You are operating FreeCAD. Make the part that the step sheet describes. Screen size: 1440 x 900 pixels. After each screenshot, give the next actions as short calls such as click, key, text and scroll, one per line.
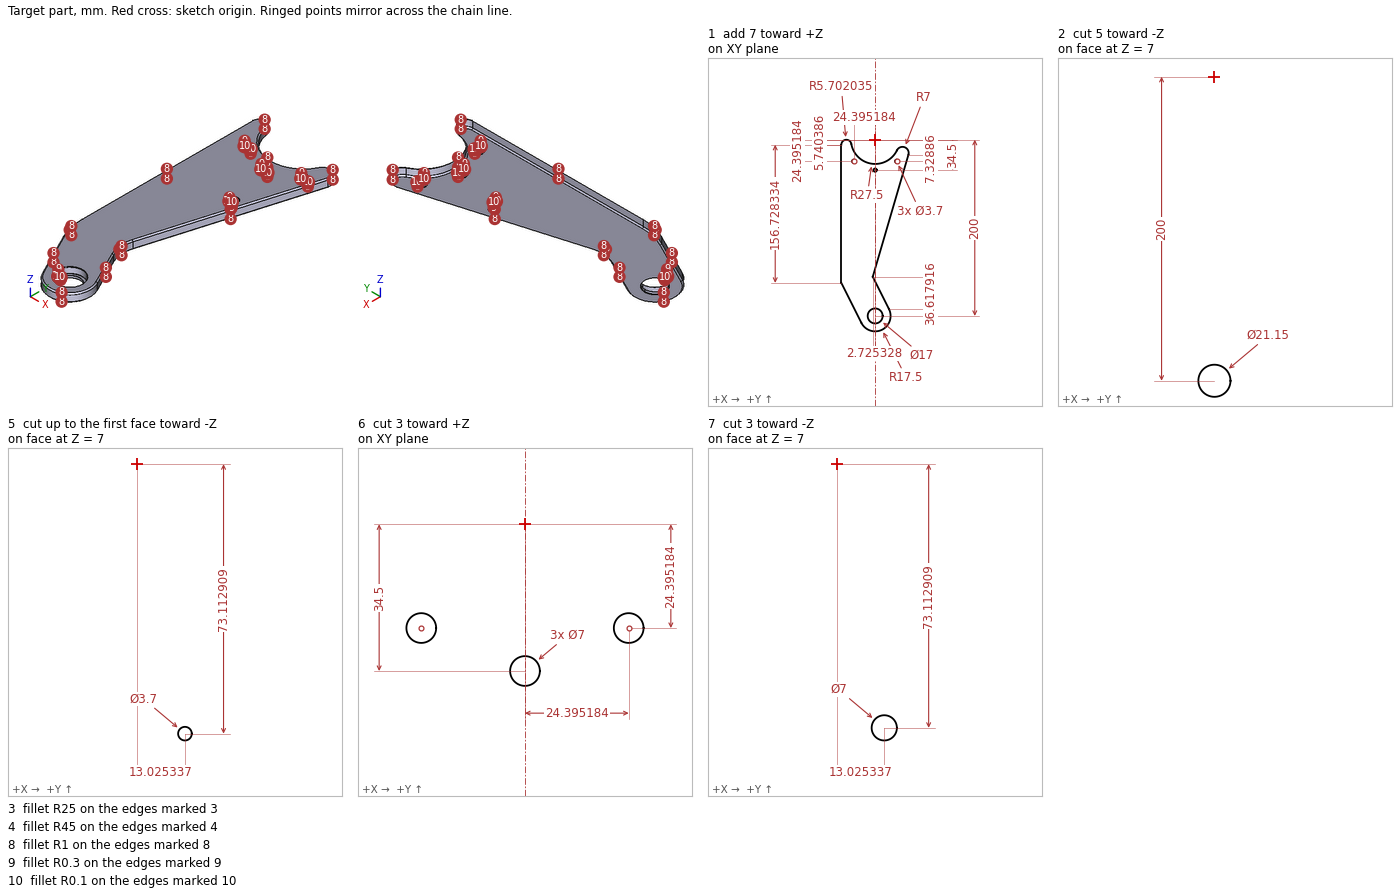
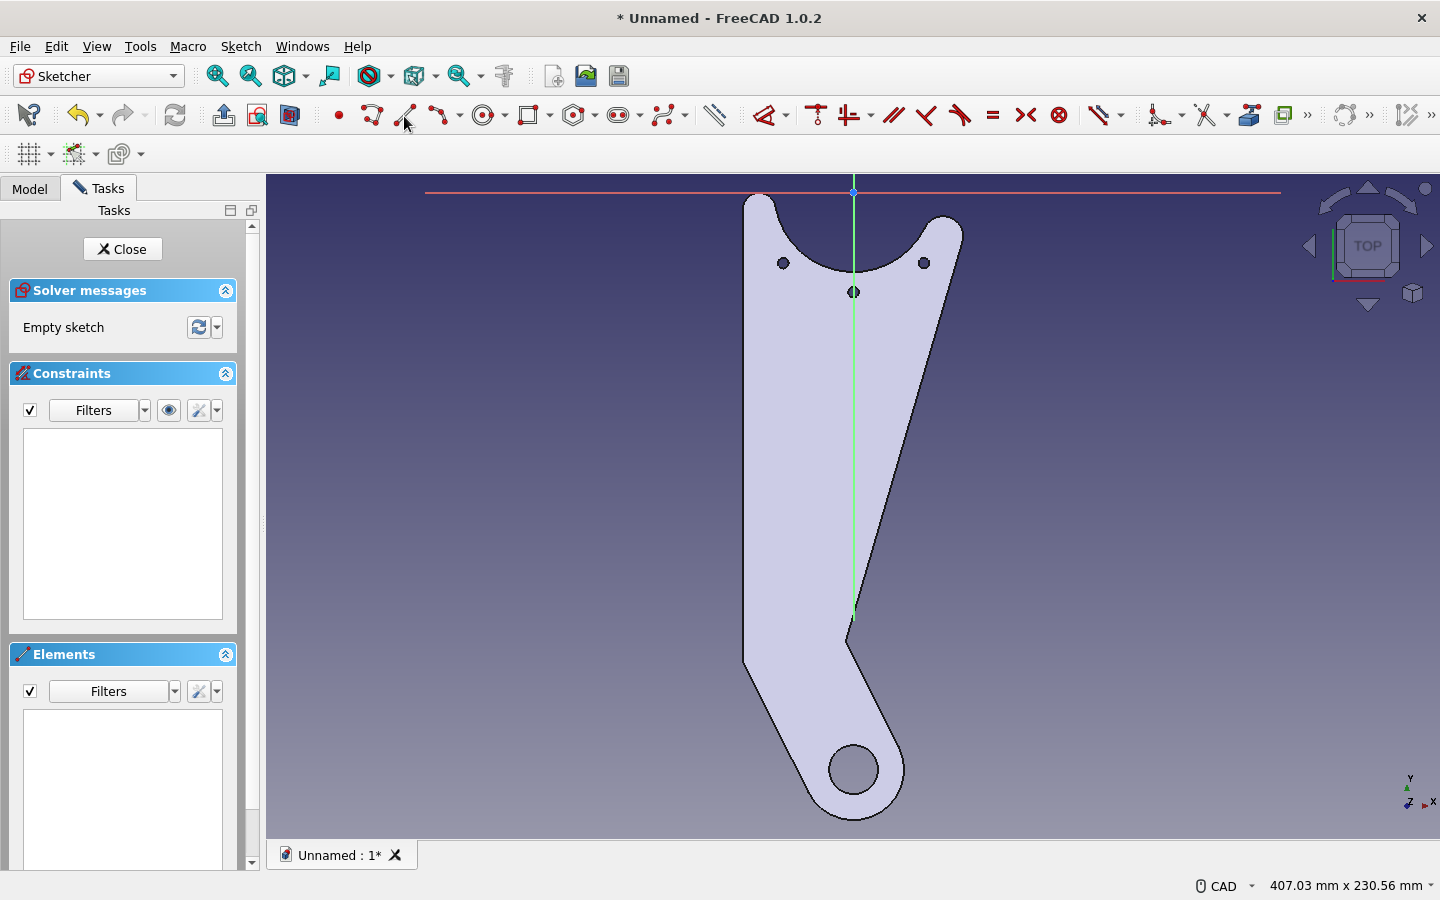
scroll(864, 811, up, 10)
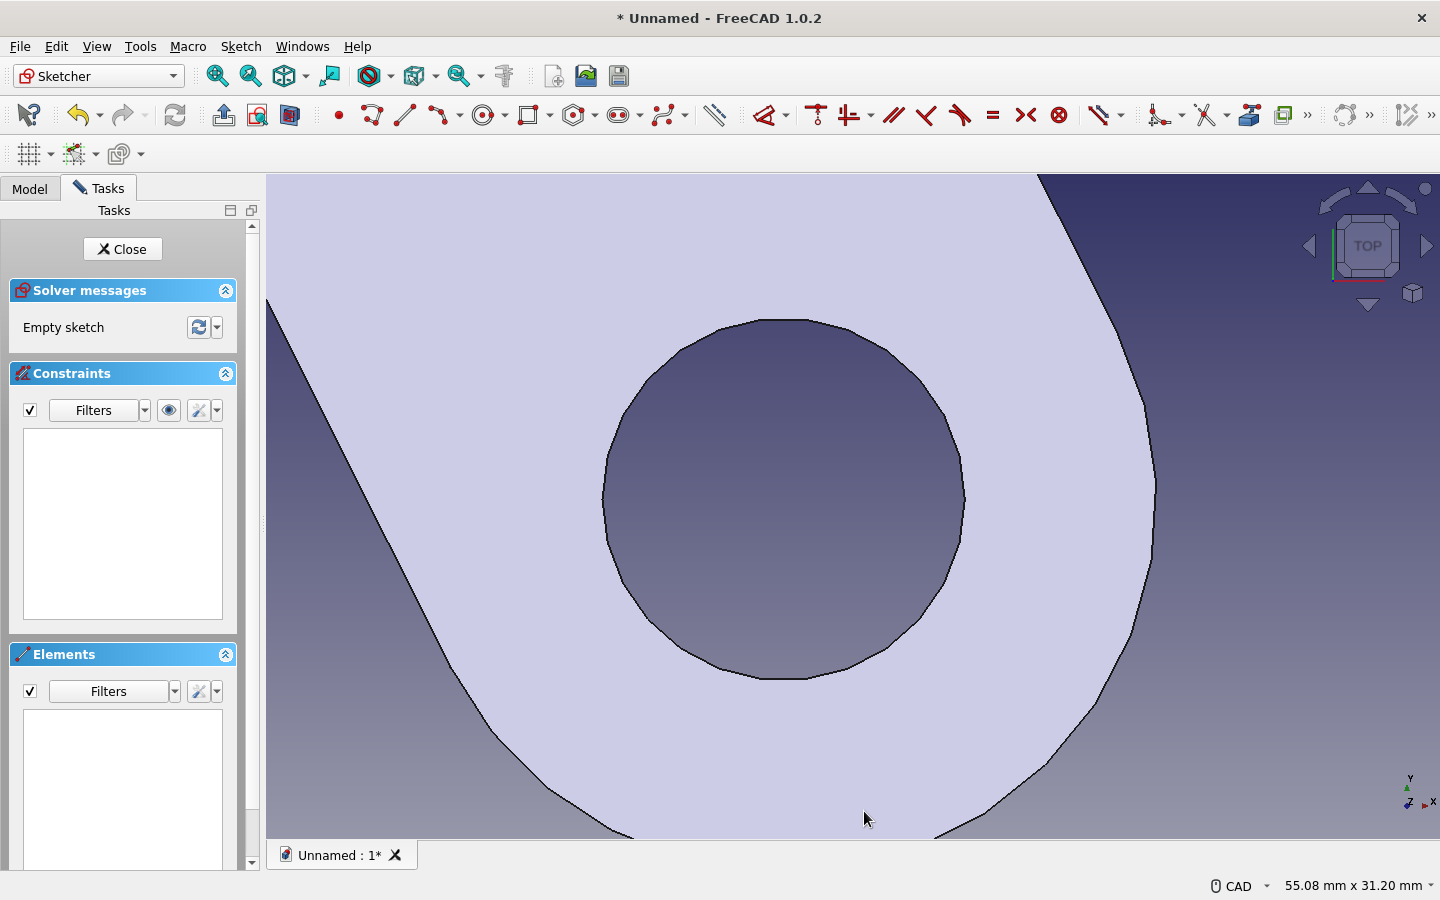
key(g)
key(c)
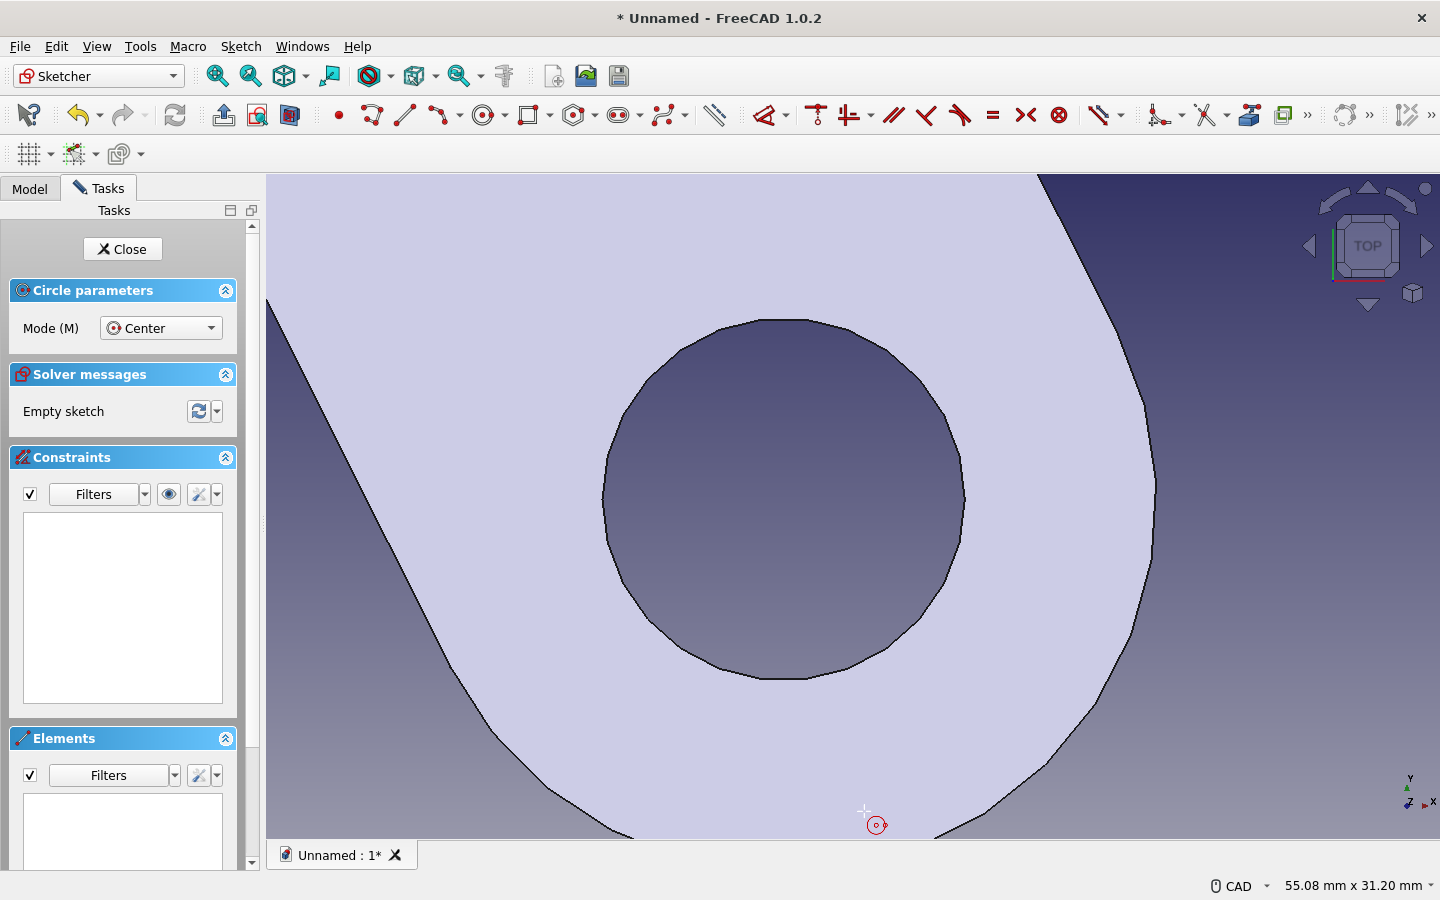
click(784, 499)
click(943, 340)
key(Escape)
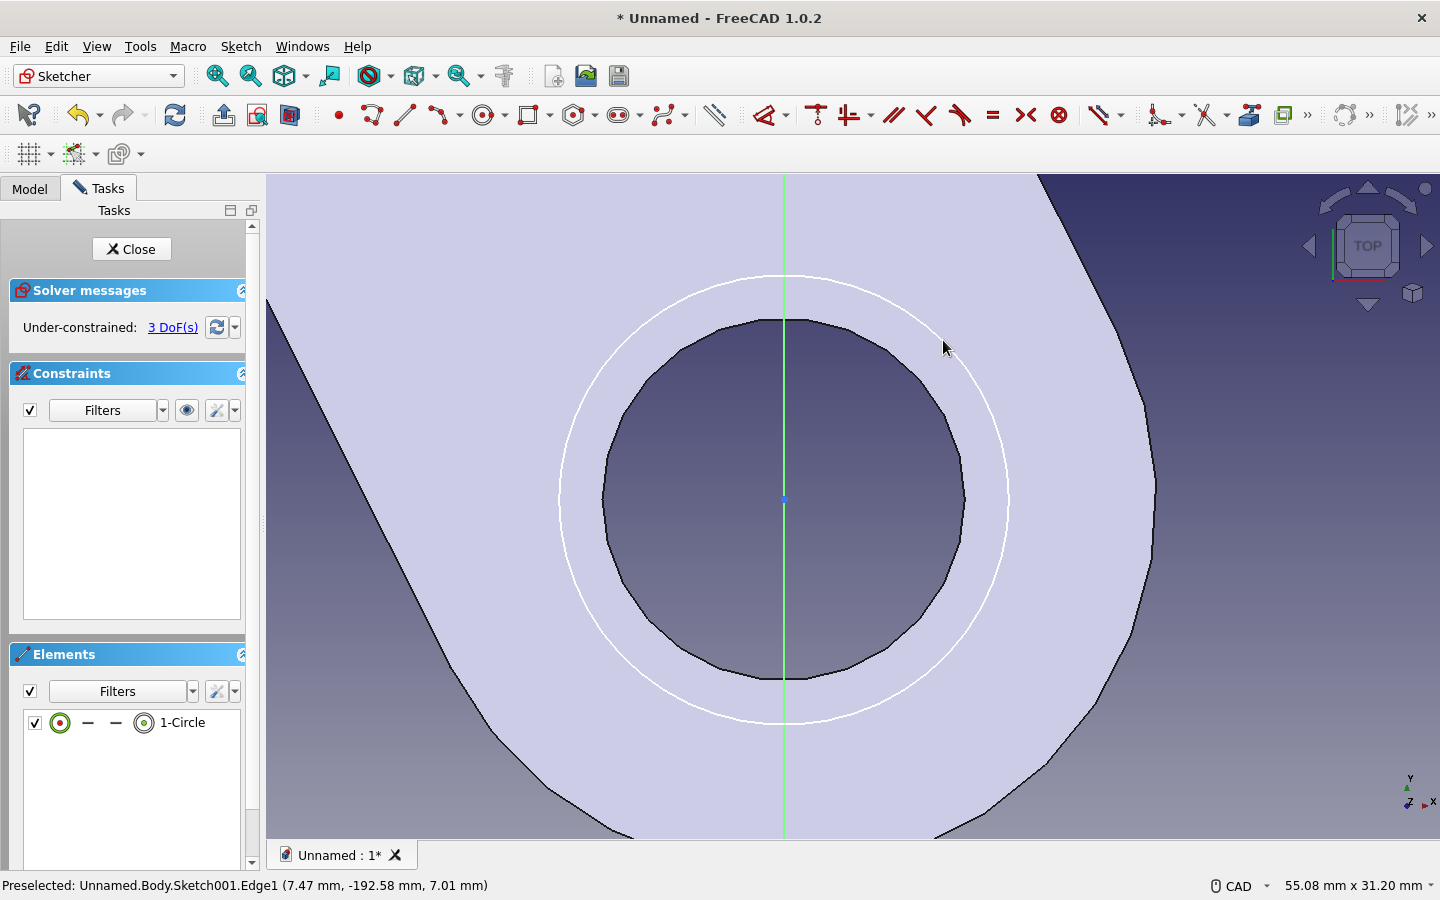
click(784, 500)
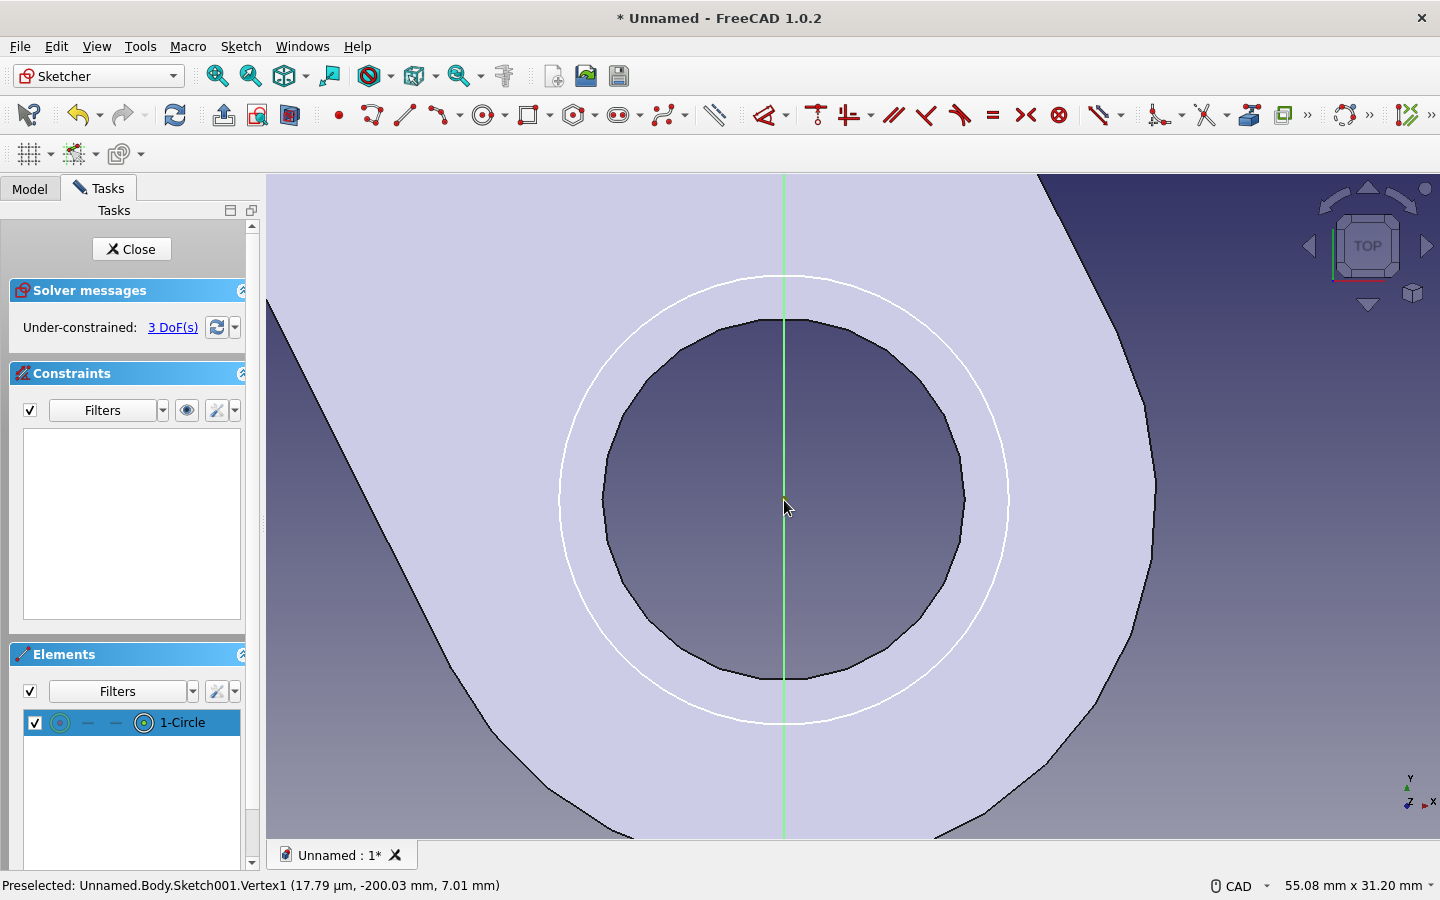
click(784, 768)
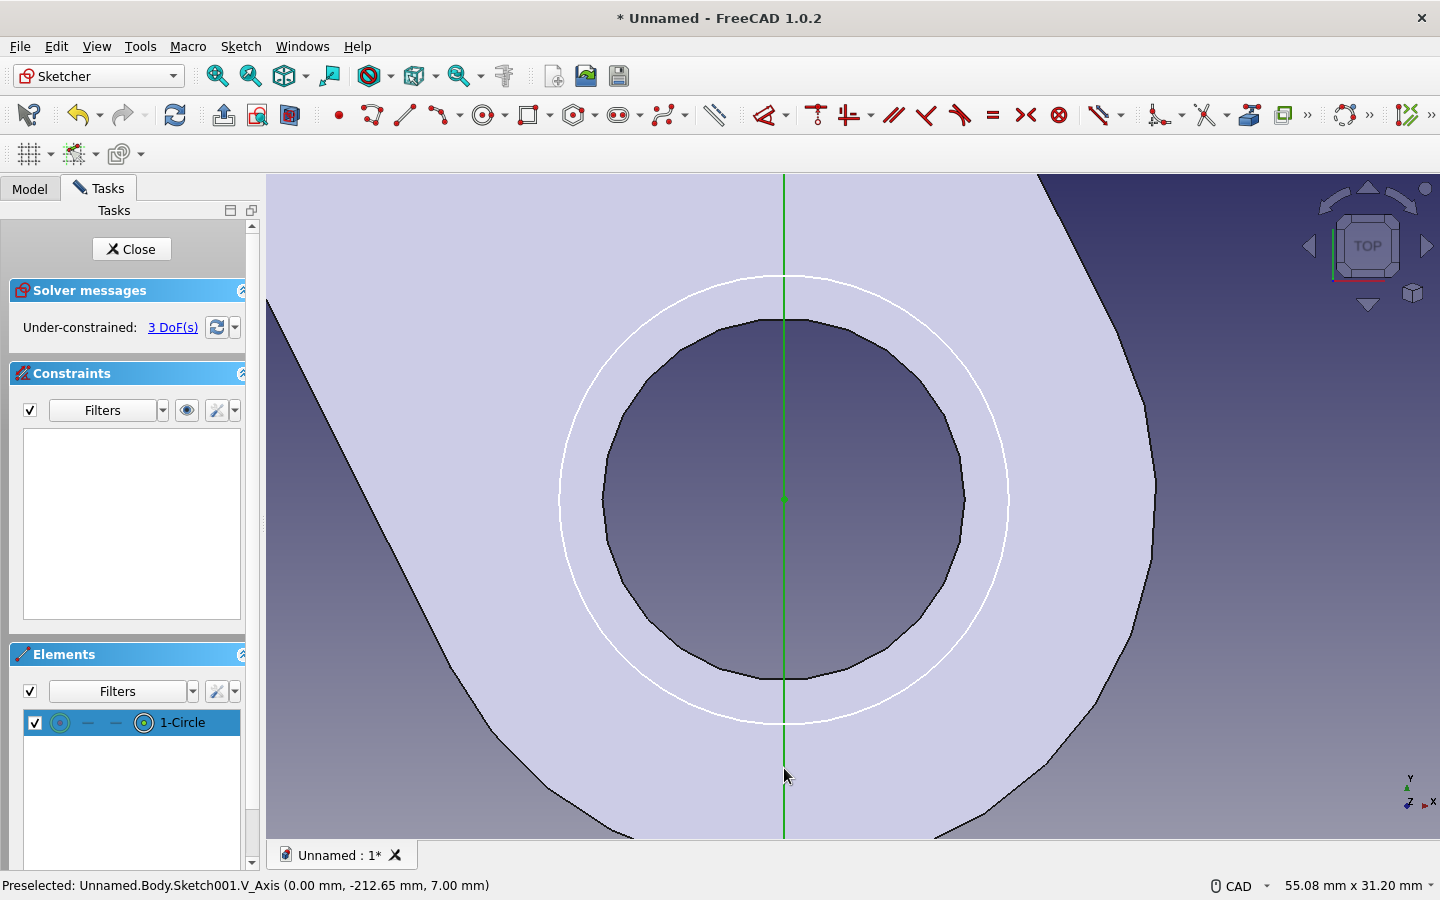
click(816, 116)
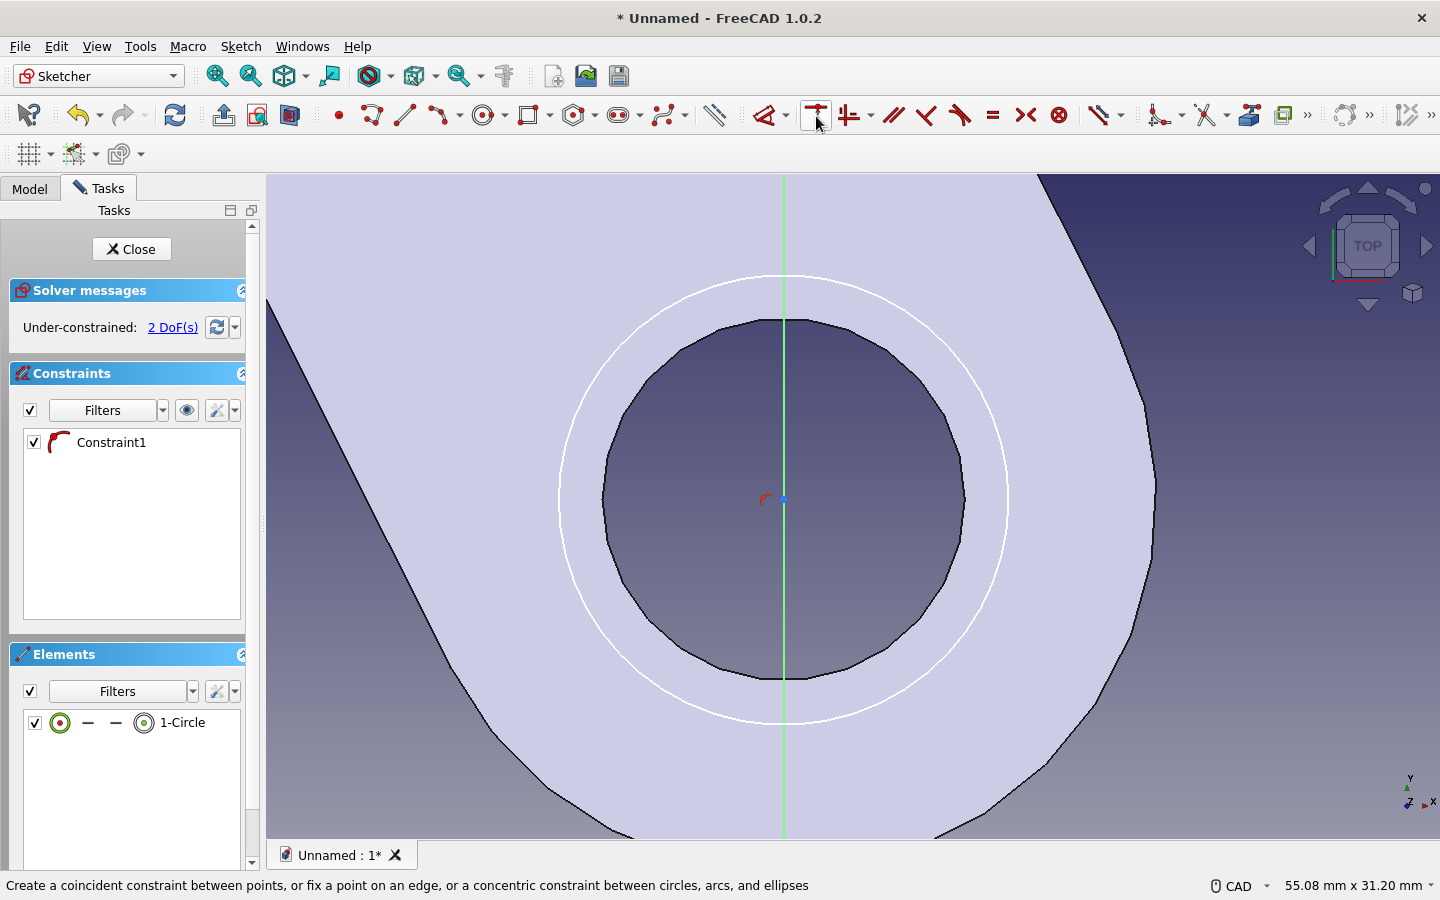
key(d)